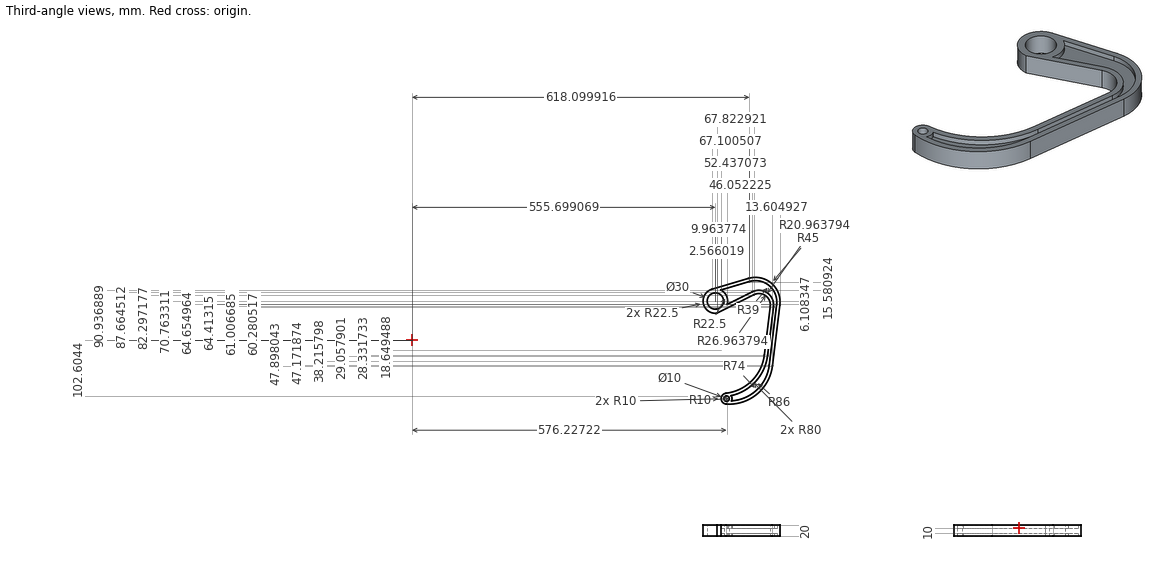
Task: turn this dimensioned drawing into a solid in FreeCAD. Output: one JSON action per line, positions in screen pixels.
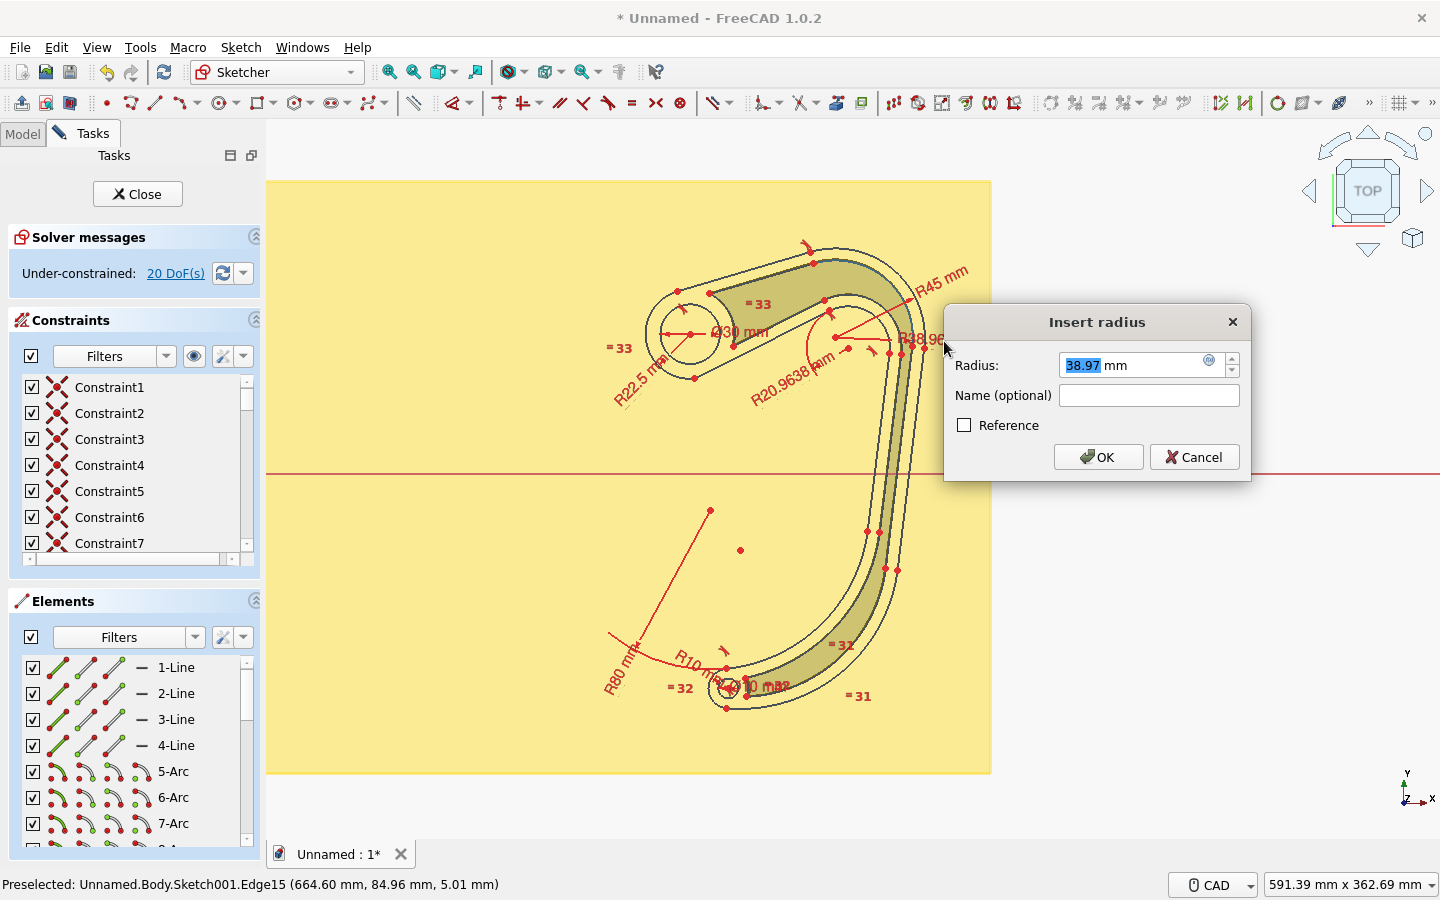
{"action": "type", "text": "39"}
{"action": "key", "text": "Return"}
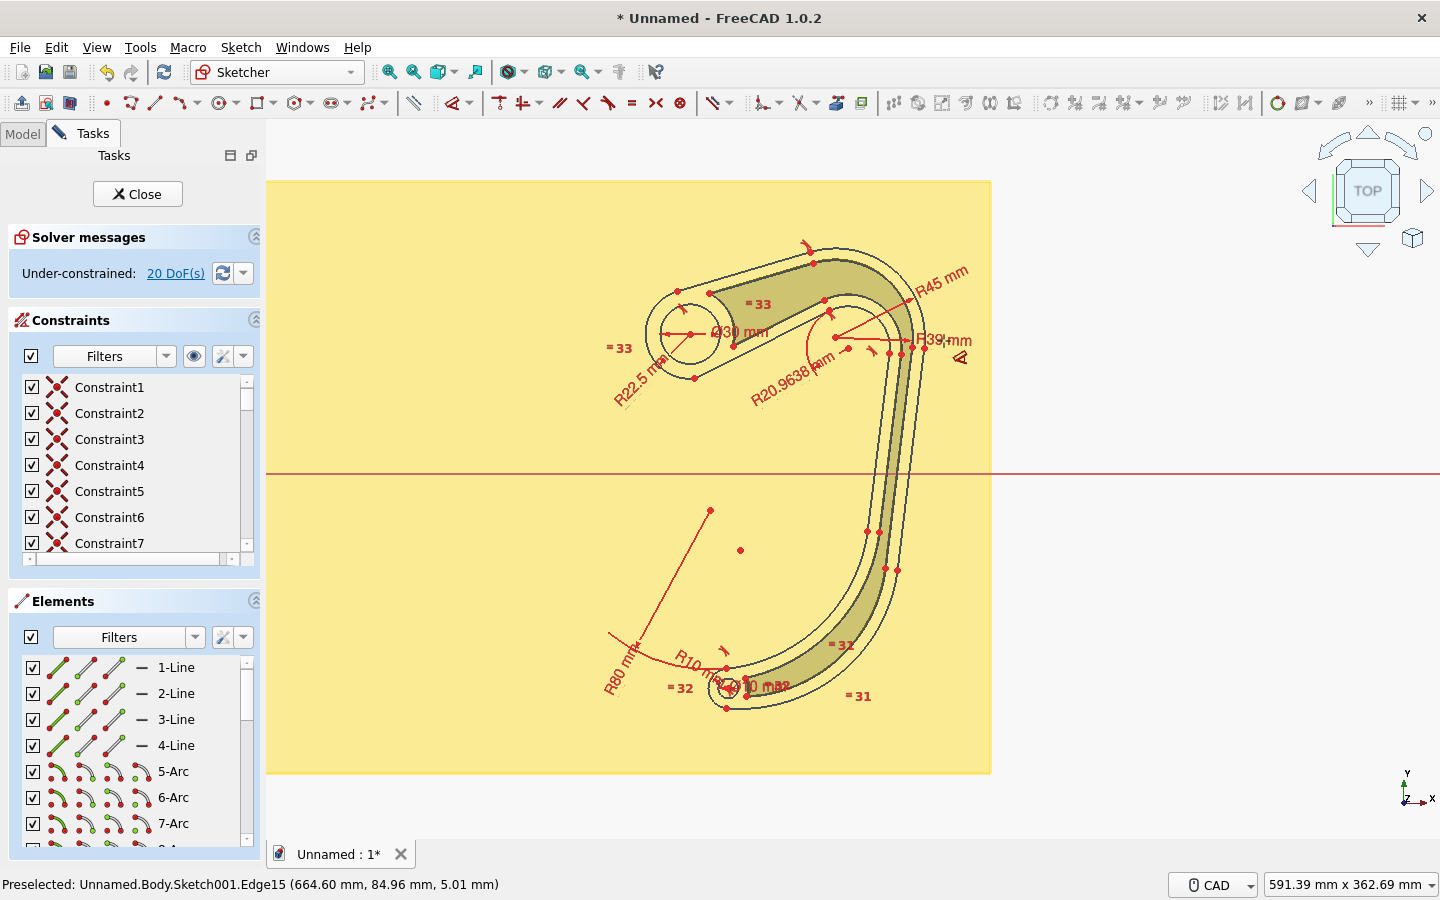
{"action": "left_click", "coordinate": [806, 681]}
{"action": "left_click", "coordinate": [820, 710]}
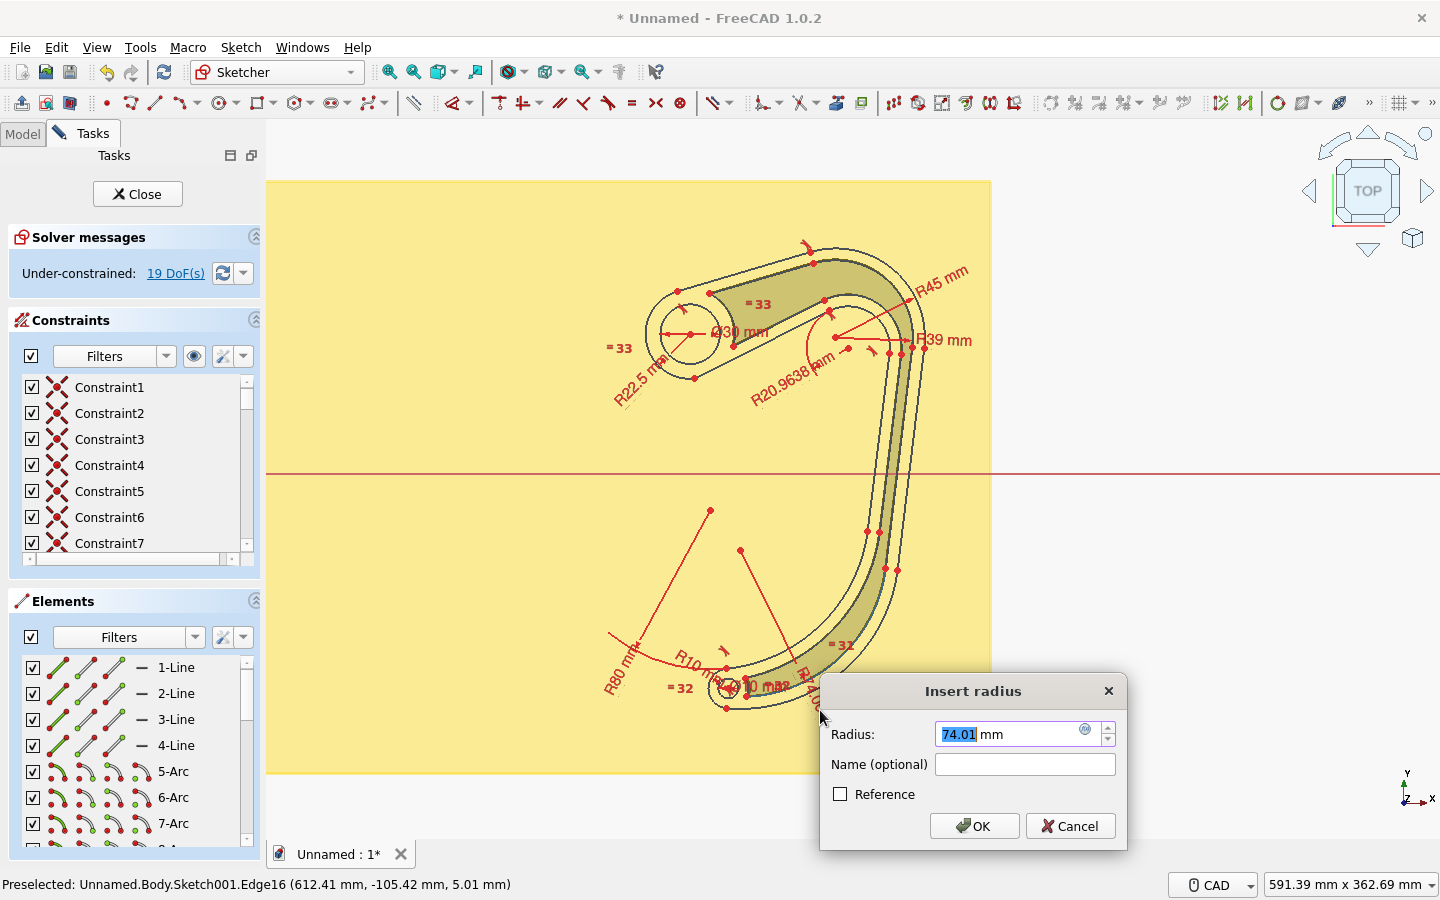
{"action": "type", "text": "74"}
{"action": "key", "text": "Return"}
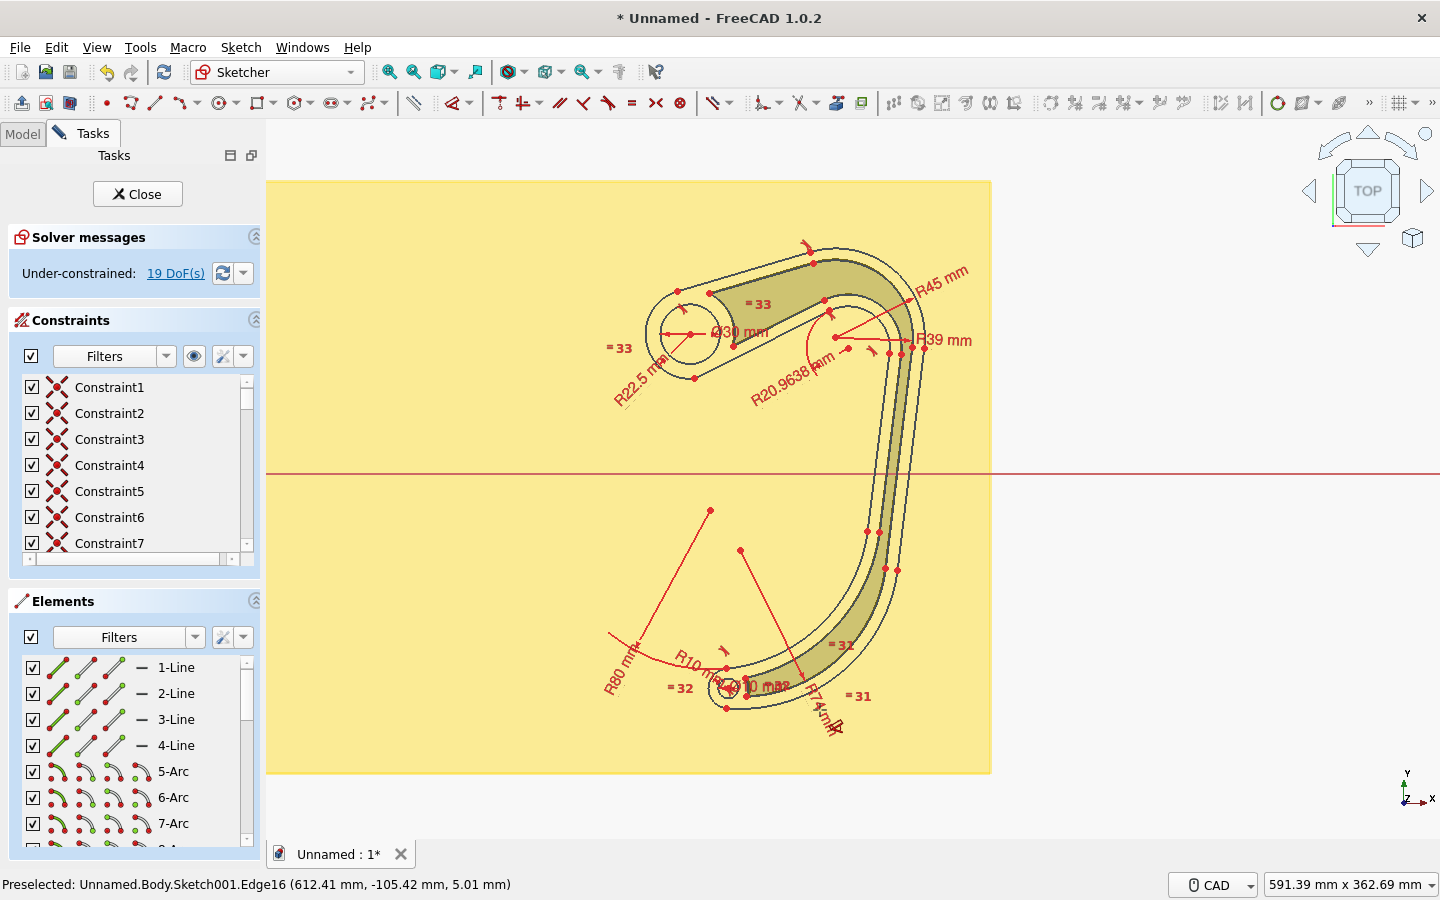
{"action": "left_click", "coordinate": [804, 654]}
{"action": "left_click", "coordinate": [627, 696]}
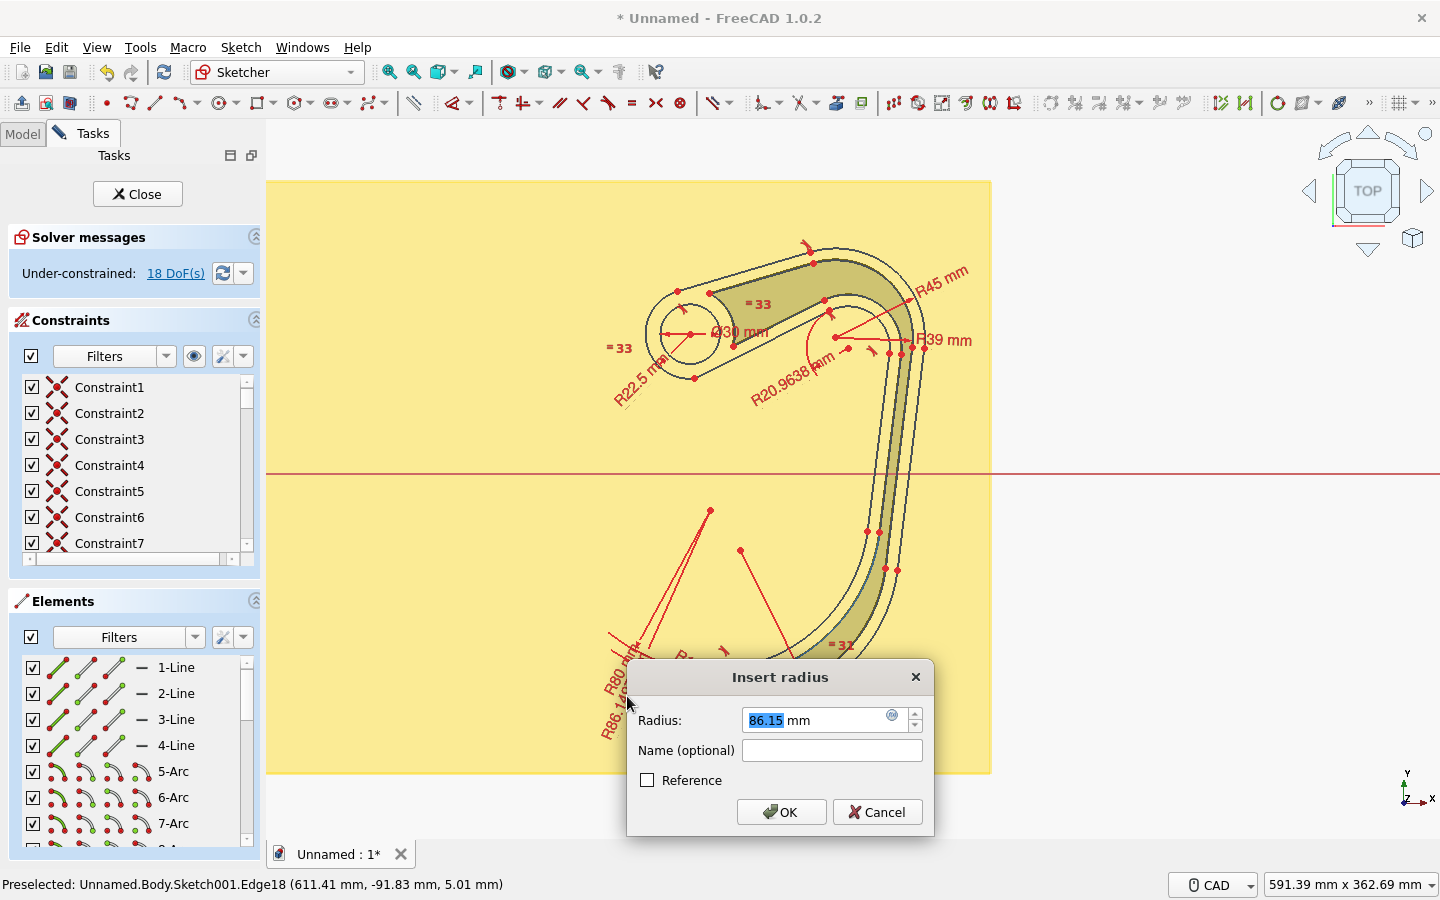
{"action": "type", "text": "86"}
{"action": "key", "text": "Return"}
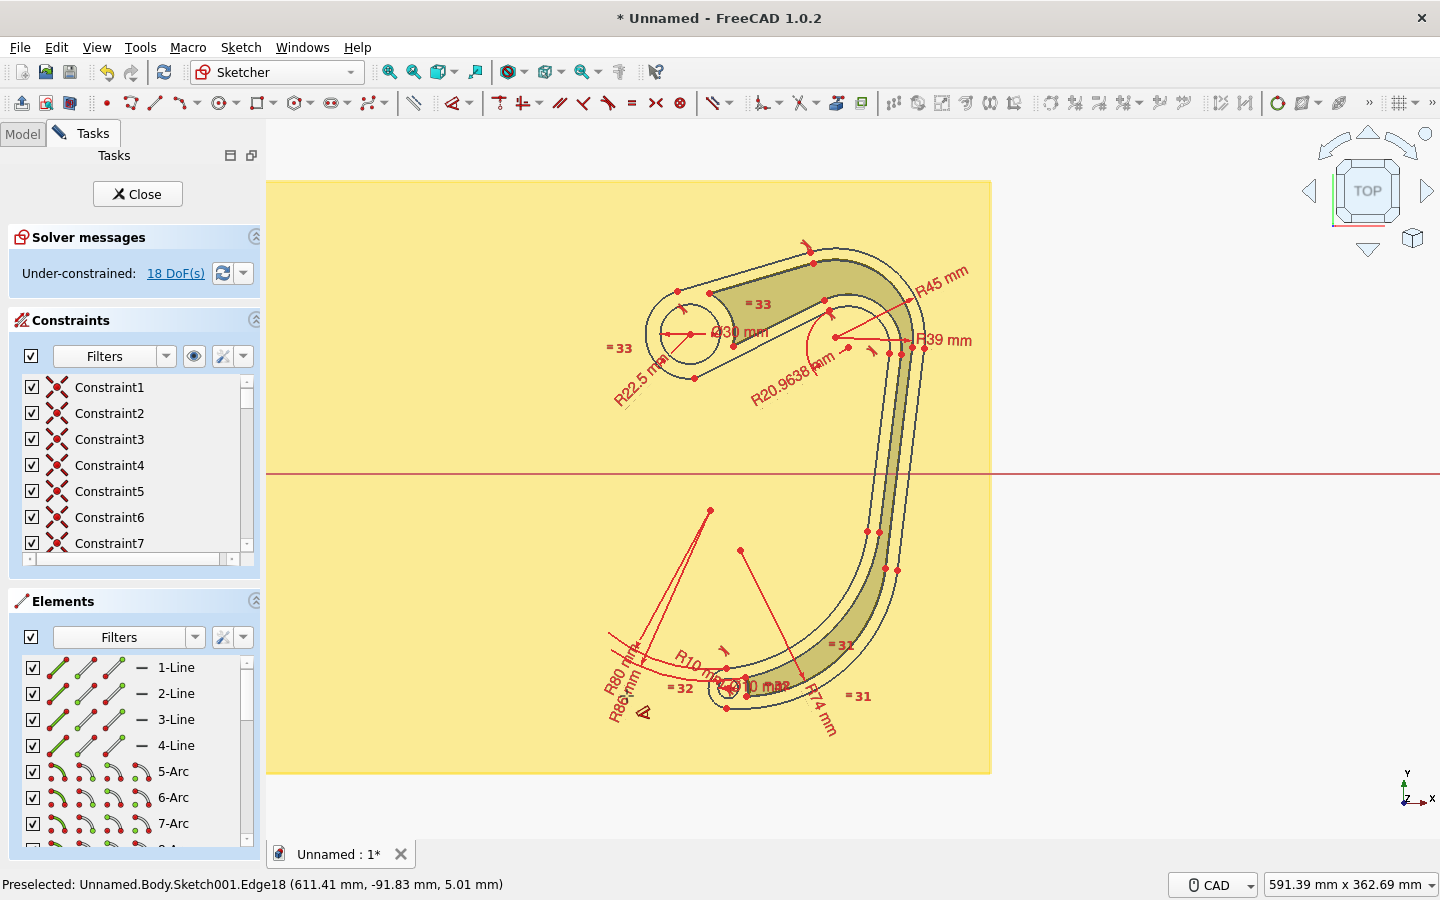
{"action": "left_click", "coordinate": [894, 321]}
{"action": "left_click", "coordinate": [904, 255]}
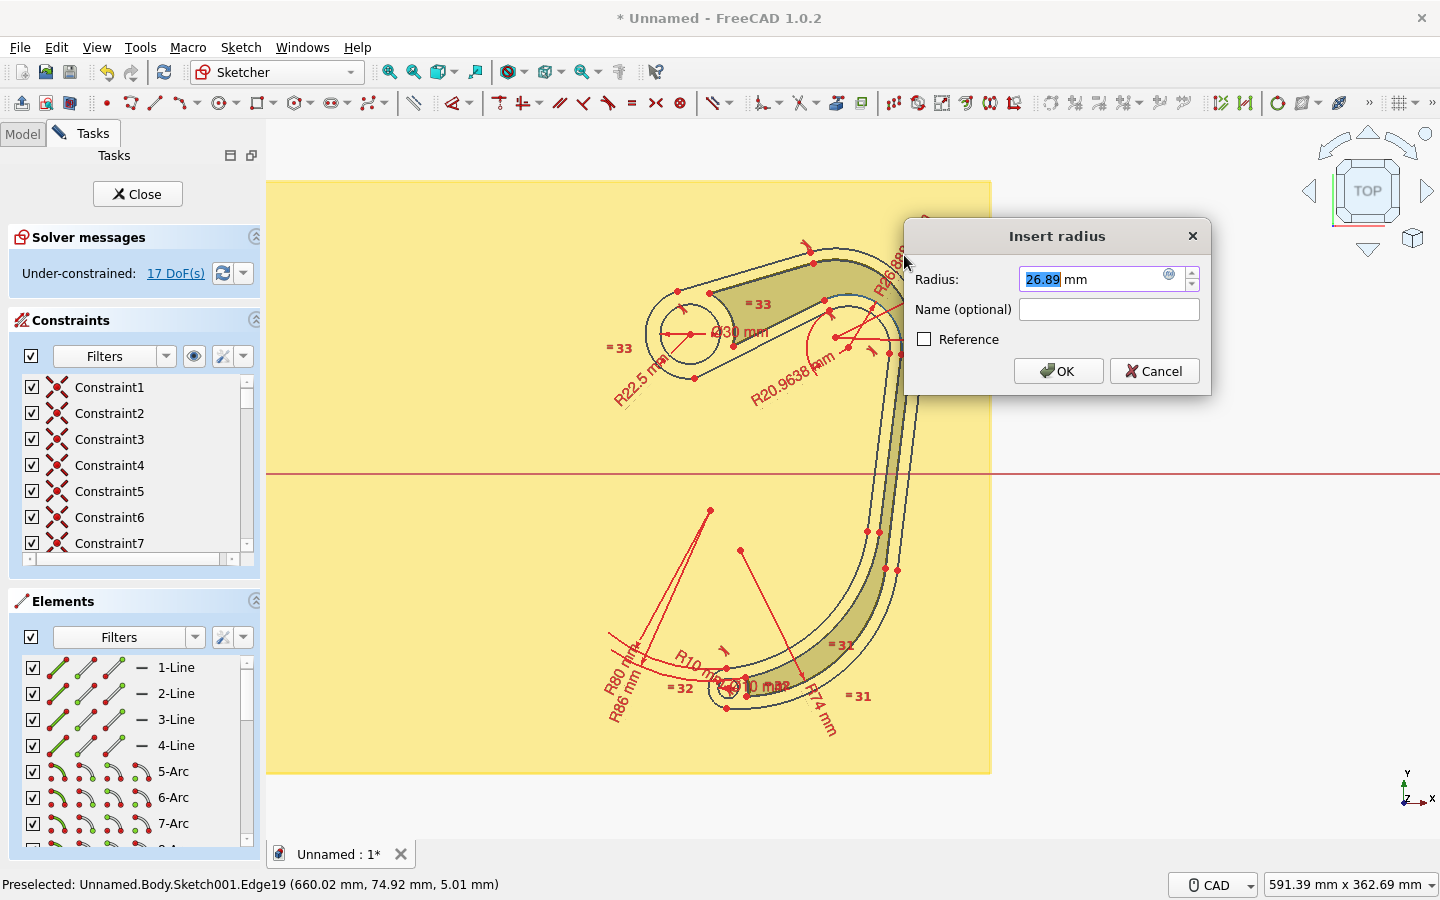
{"action": "type", "text": "26.963794"}
{"action": "key", "text": "Return"}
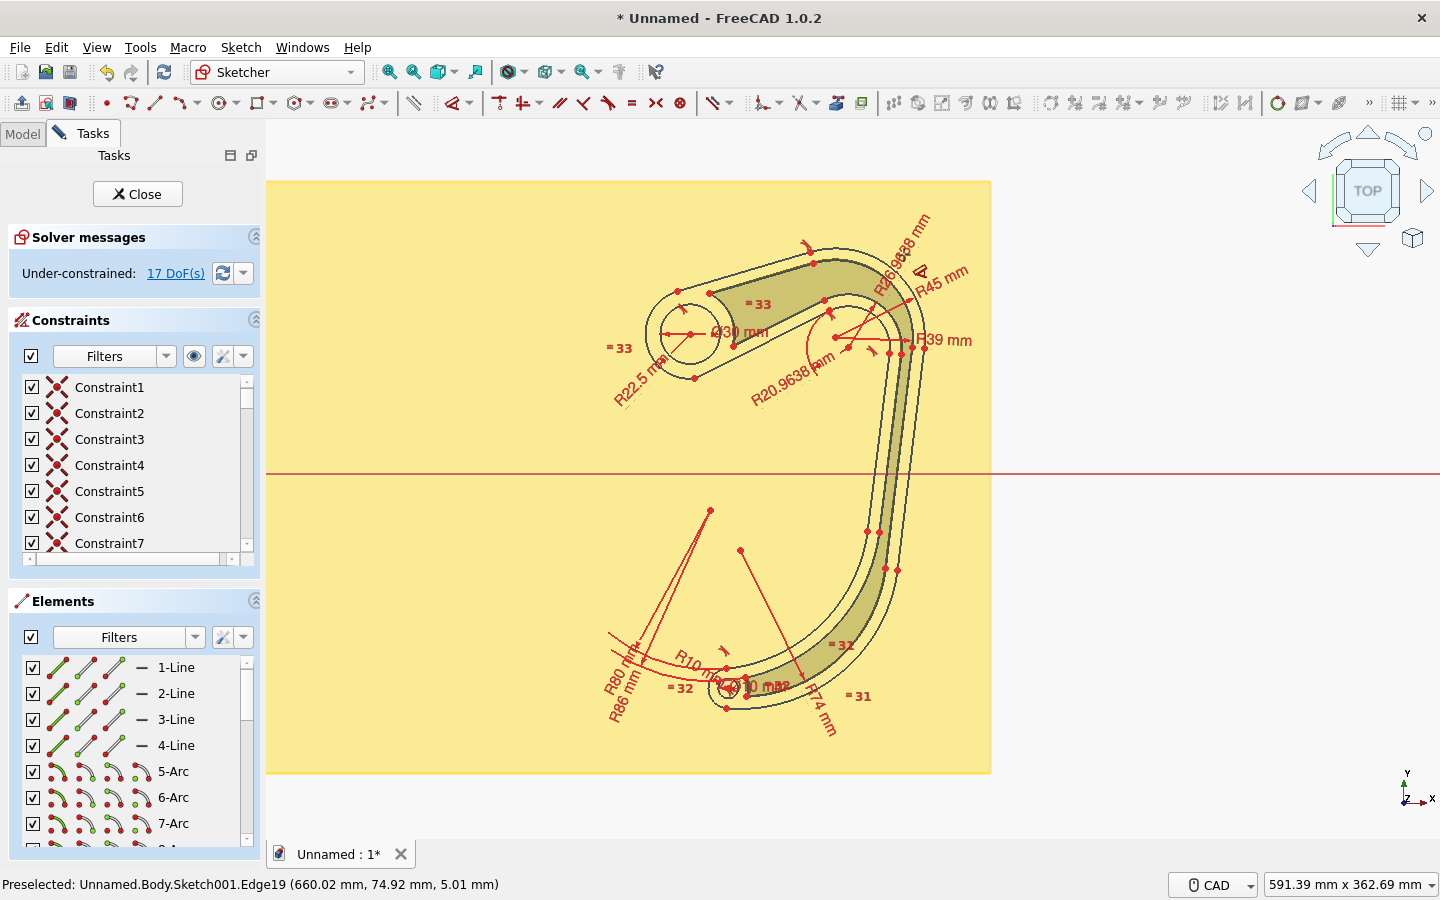
{"action": "left_click", "coordinate": [912, 347]}
{"action": "left_click", "coordinate": [946, 410]}